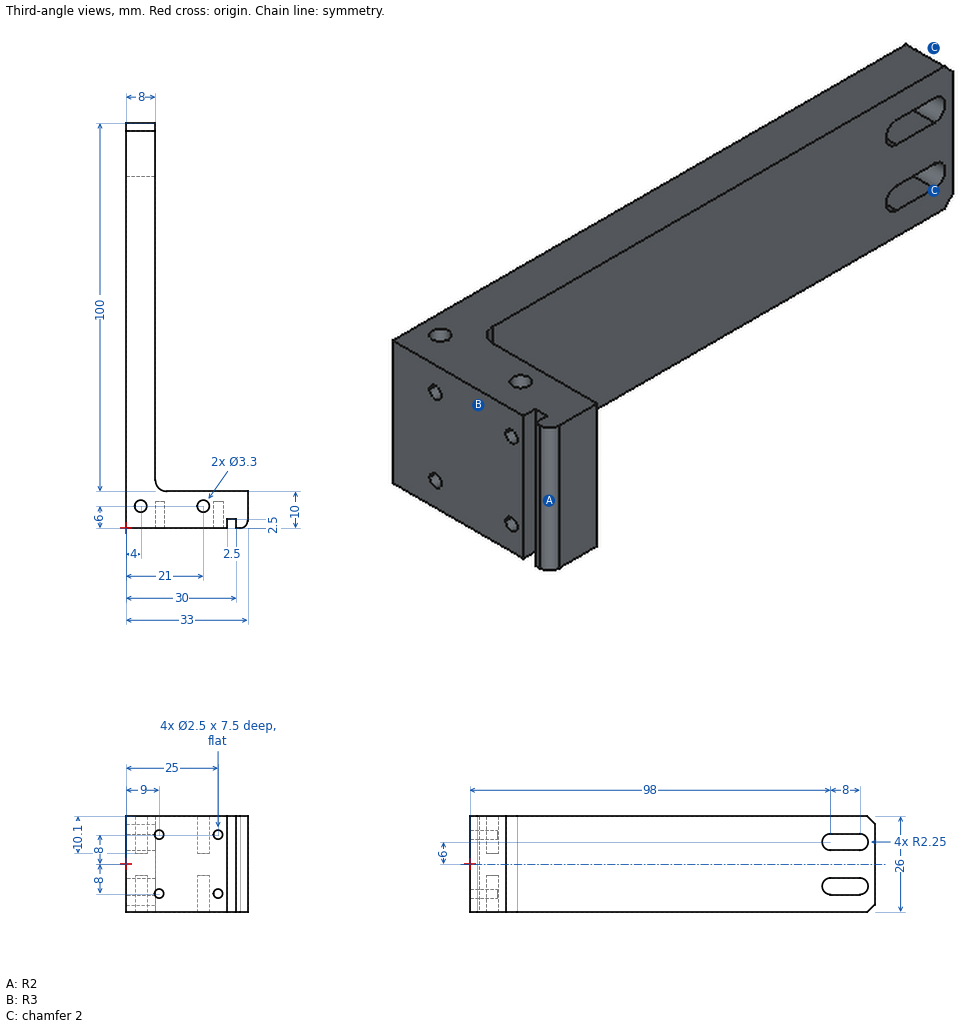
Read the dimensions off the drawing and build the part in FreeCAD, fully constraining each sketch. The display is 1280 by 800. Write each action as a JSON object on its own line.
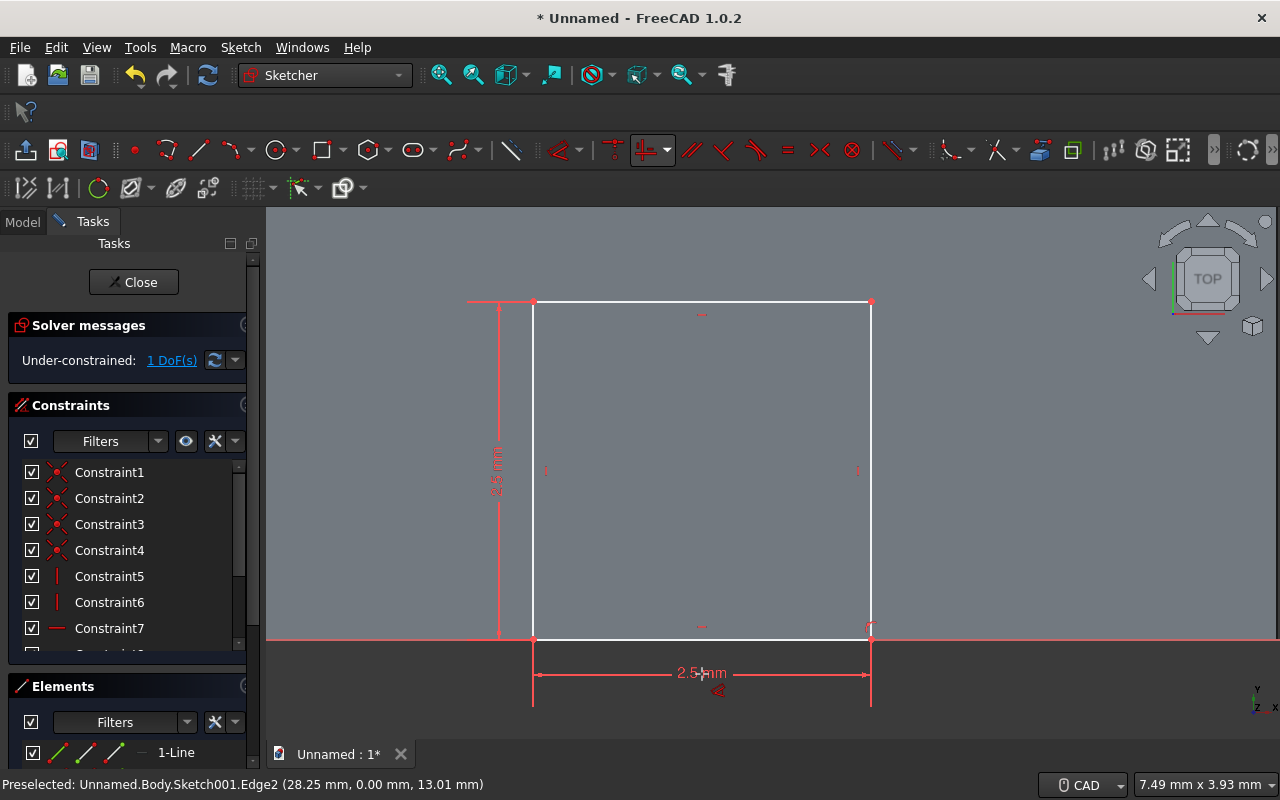
{"action": "left_click", "coordinate": [871, 640]}
{"action": "left_click", "coordinate": [583, 674]}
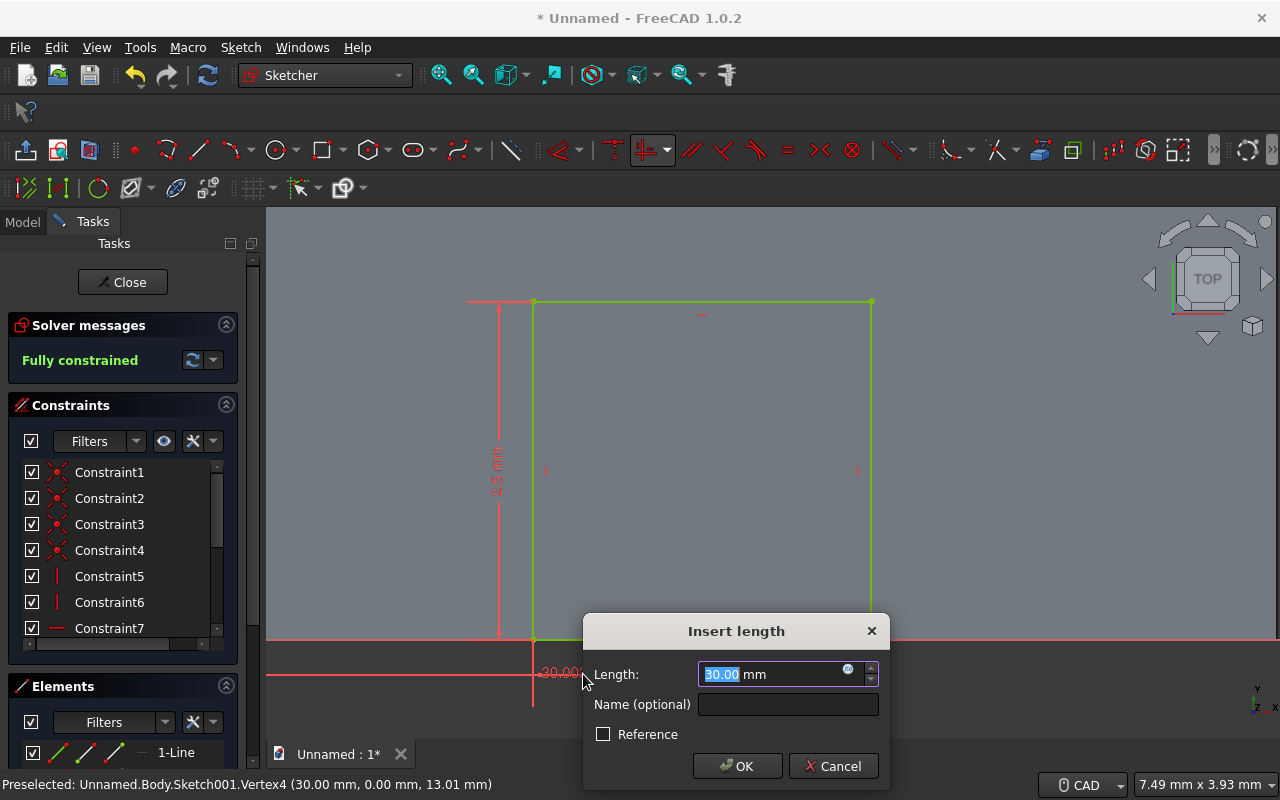
{"action": "type", "text": "30"}
{"action": "key", "text": "Return"}
{"action": "key", "text": "Escape"}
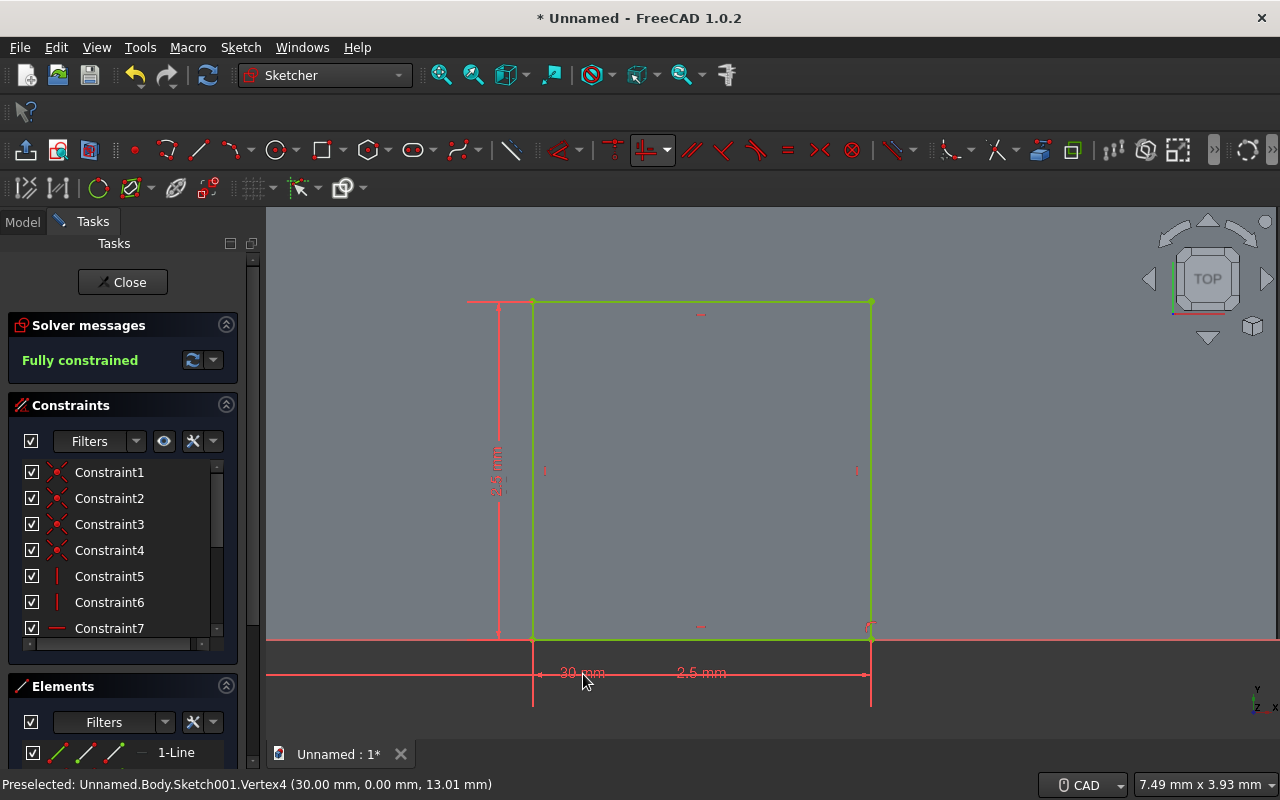
{"action": "left_click", "coordinate": [123, 282]}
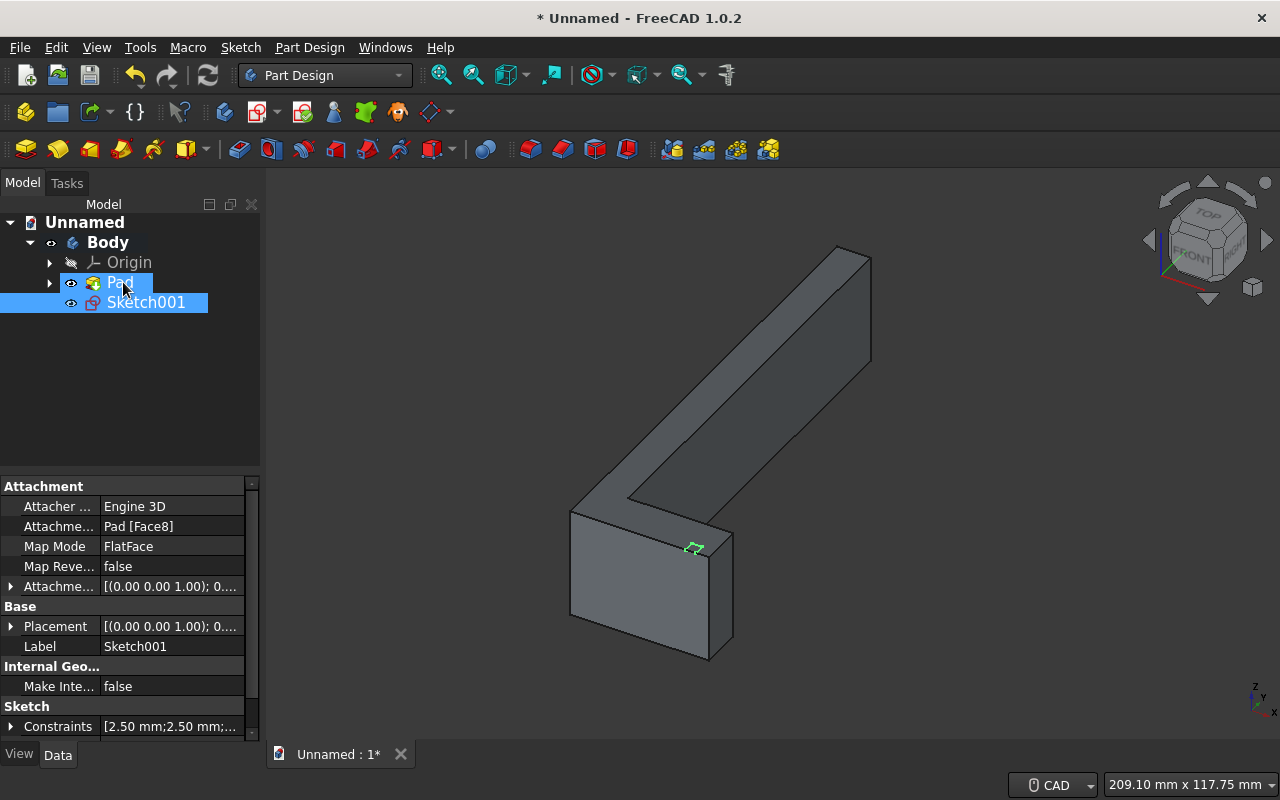
{"action": "left_click", "coordinate": [240, 150]}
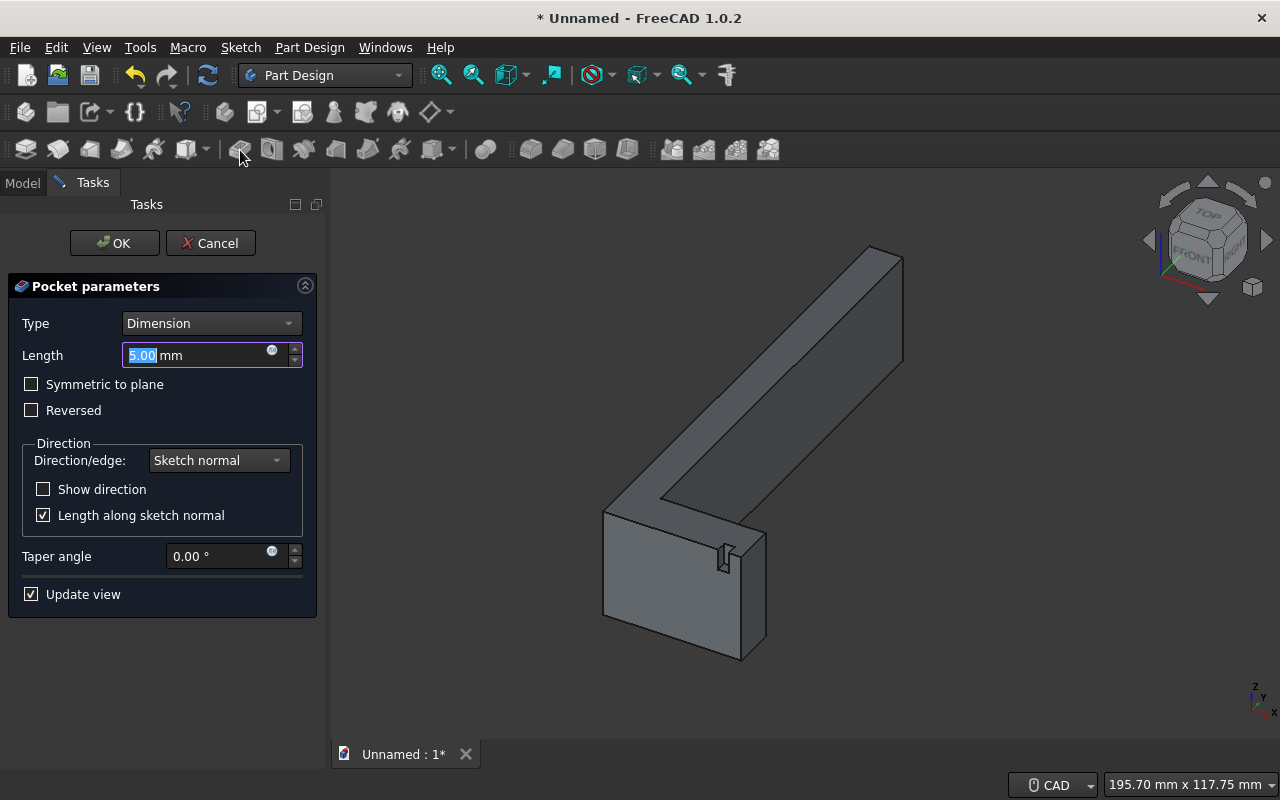
{"action": "left_click", "coordinate": [212, 324]}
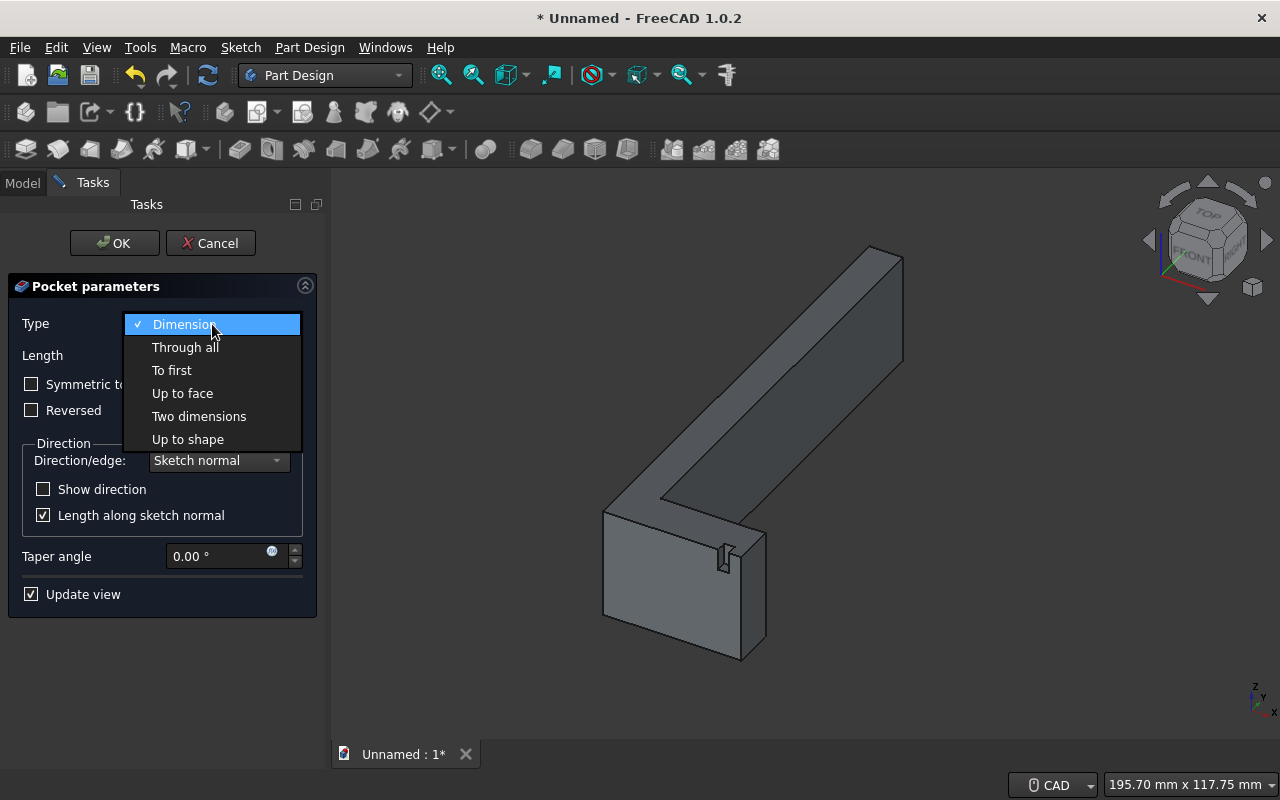
{"action": "left_click", "coordinate": [212, 348]}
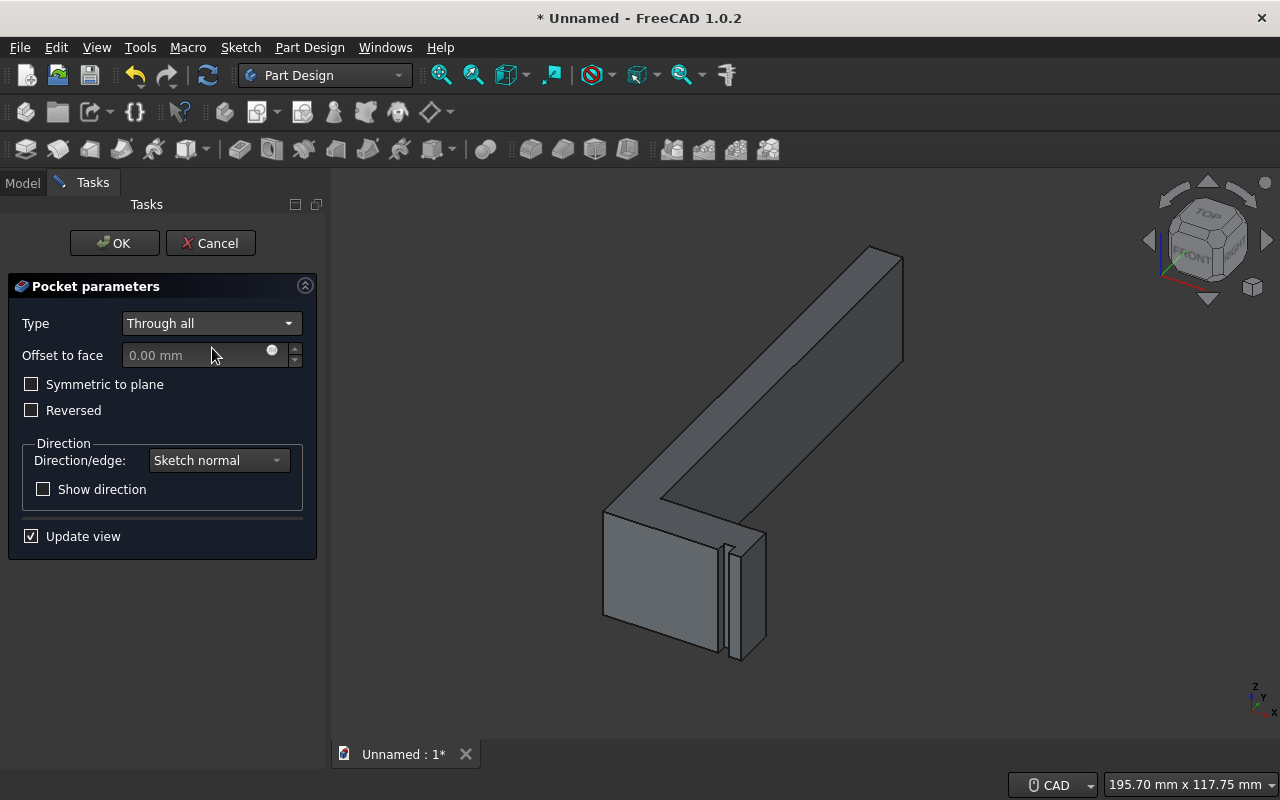
{"action": "left_click", "coordinate": [115, 243]}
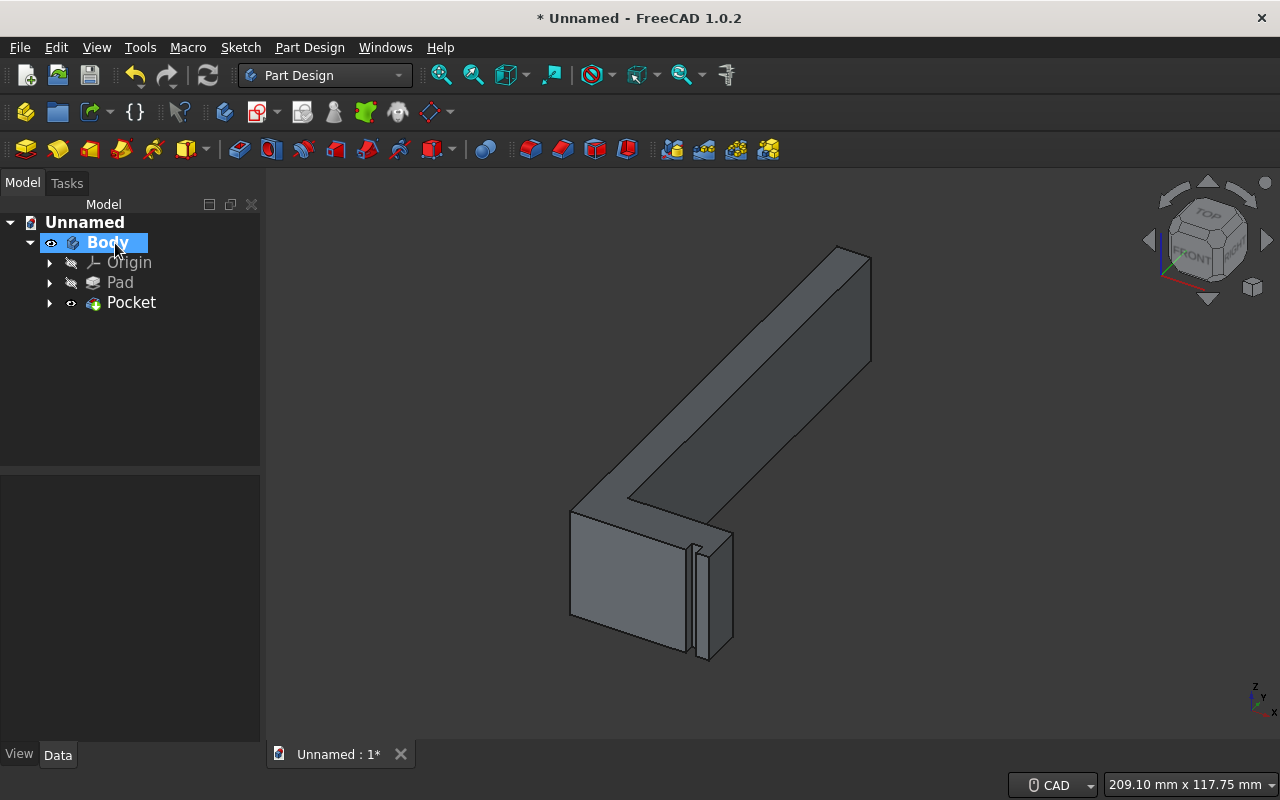
{"action": "left_click", "coordinate": [828, 268]}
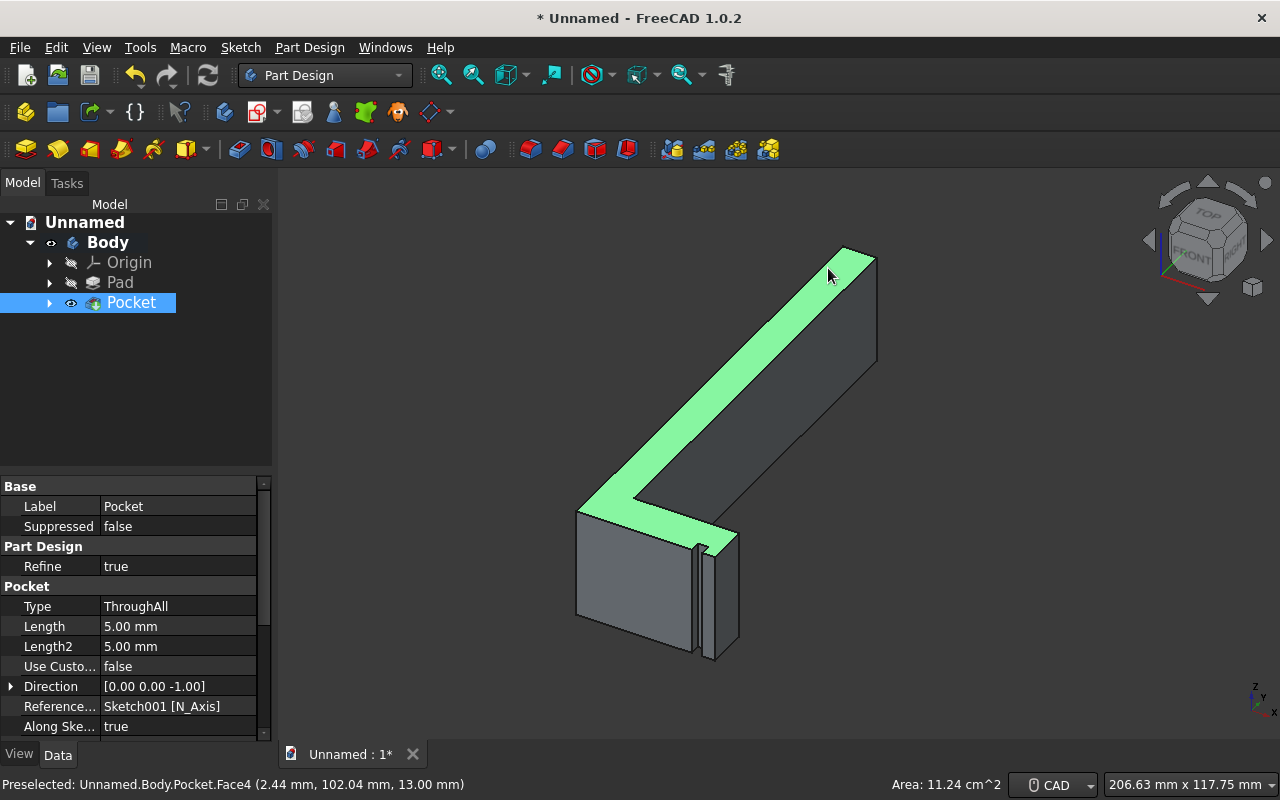
{"action": "left_click", "coordinate": [258, 112]}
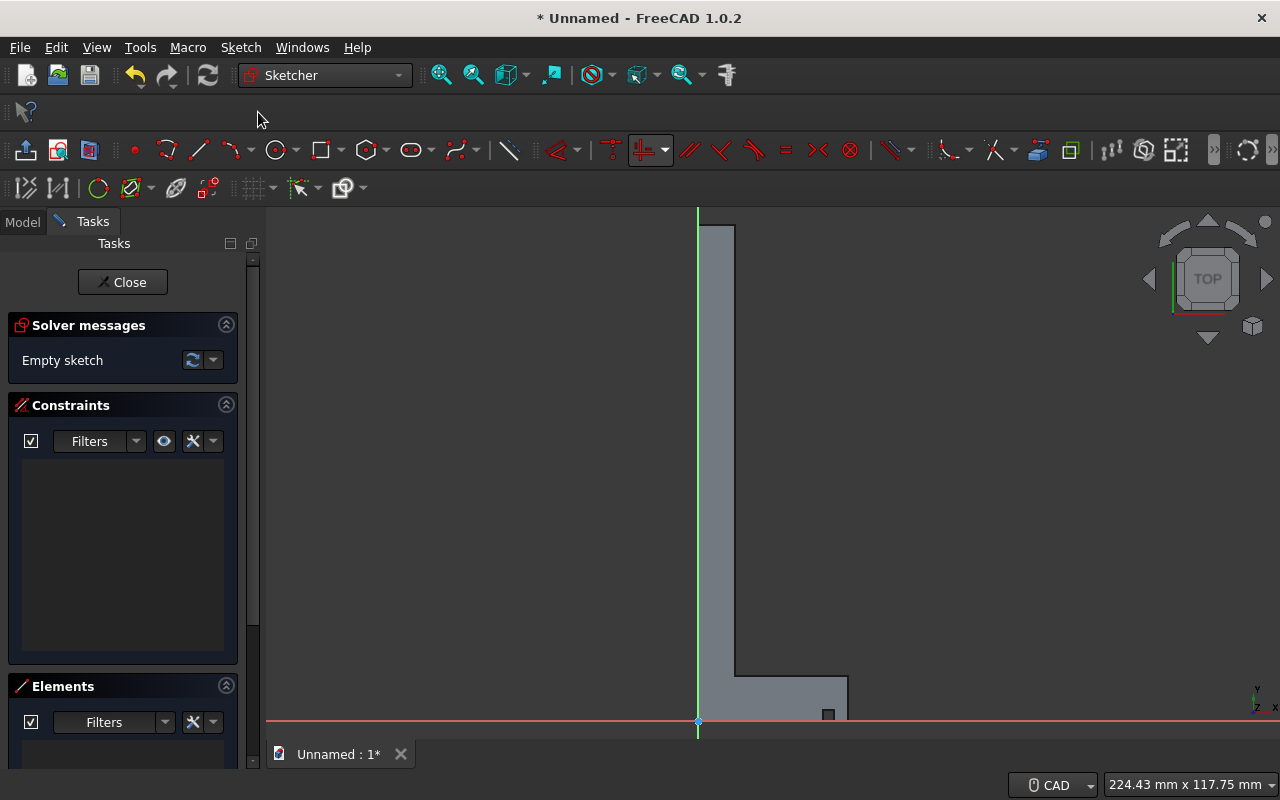
{"action": "scroll", "coordinate": [704, 473], "scroll_direction": "down", "scroll_amount": 5}